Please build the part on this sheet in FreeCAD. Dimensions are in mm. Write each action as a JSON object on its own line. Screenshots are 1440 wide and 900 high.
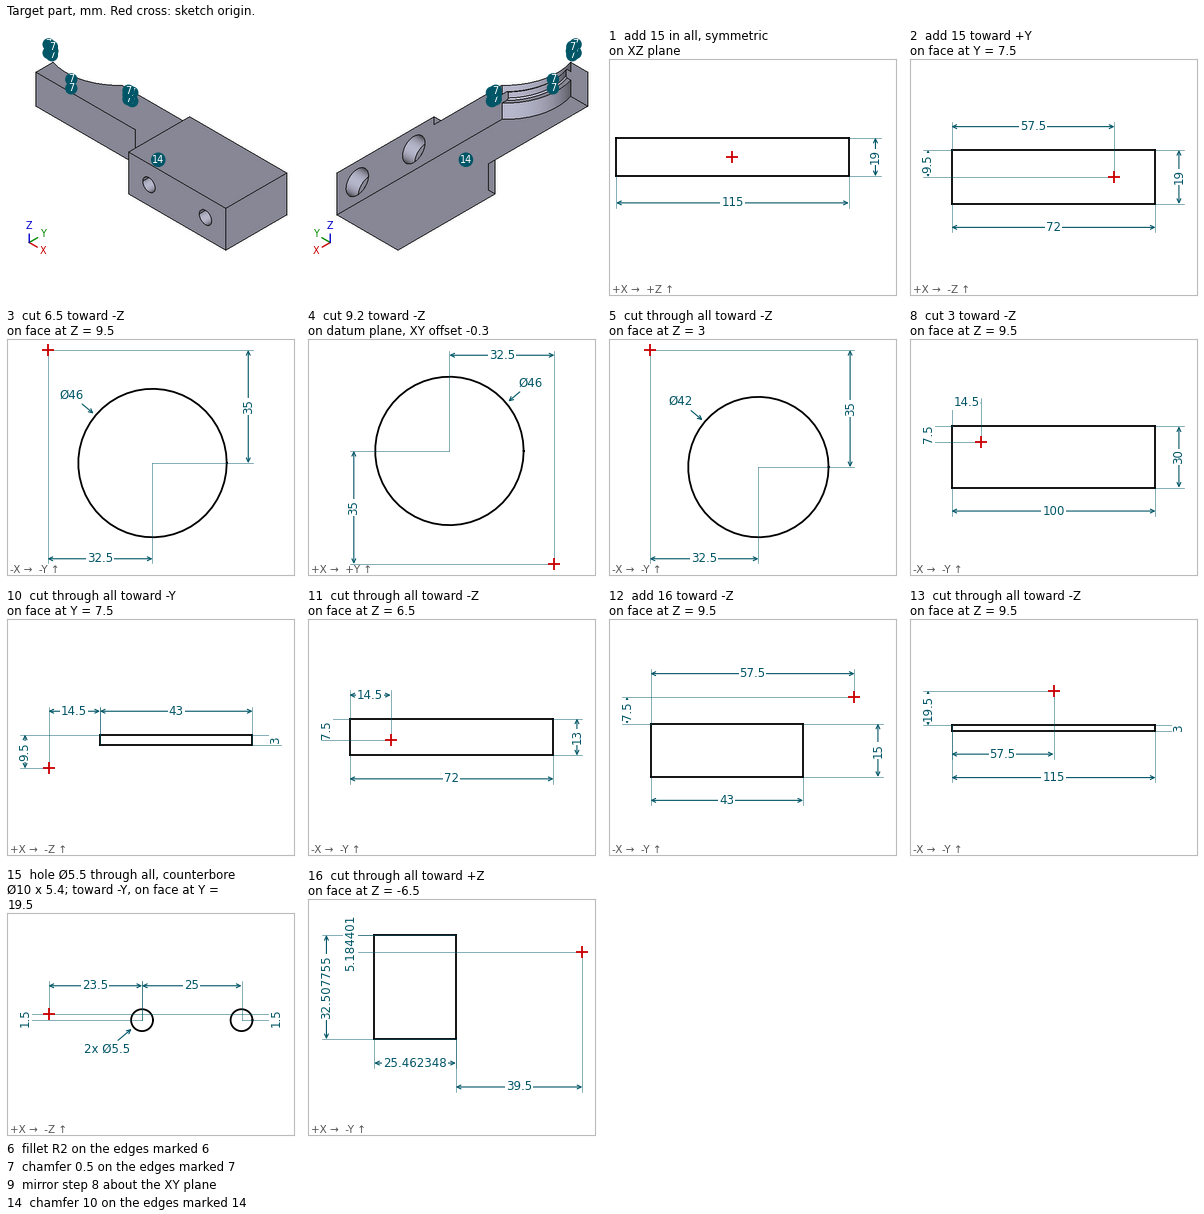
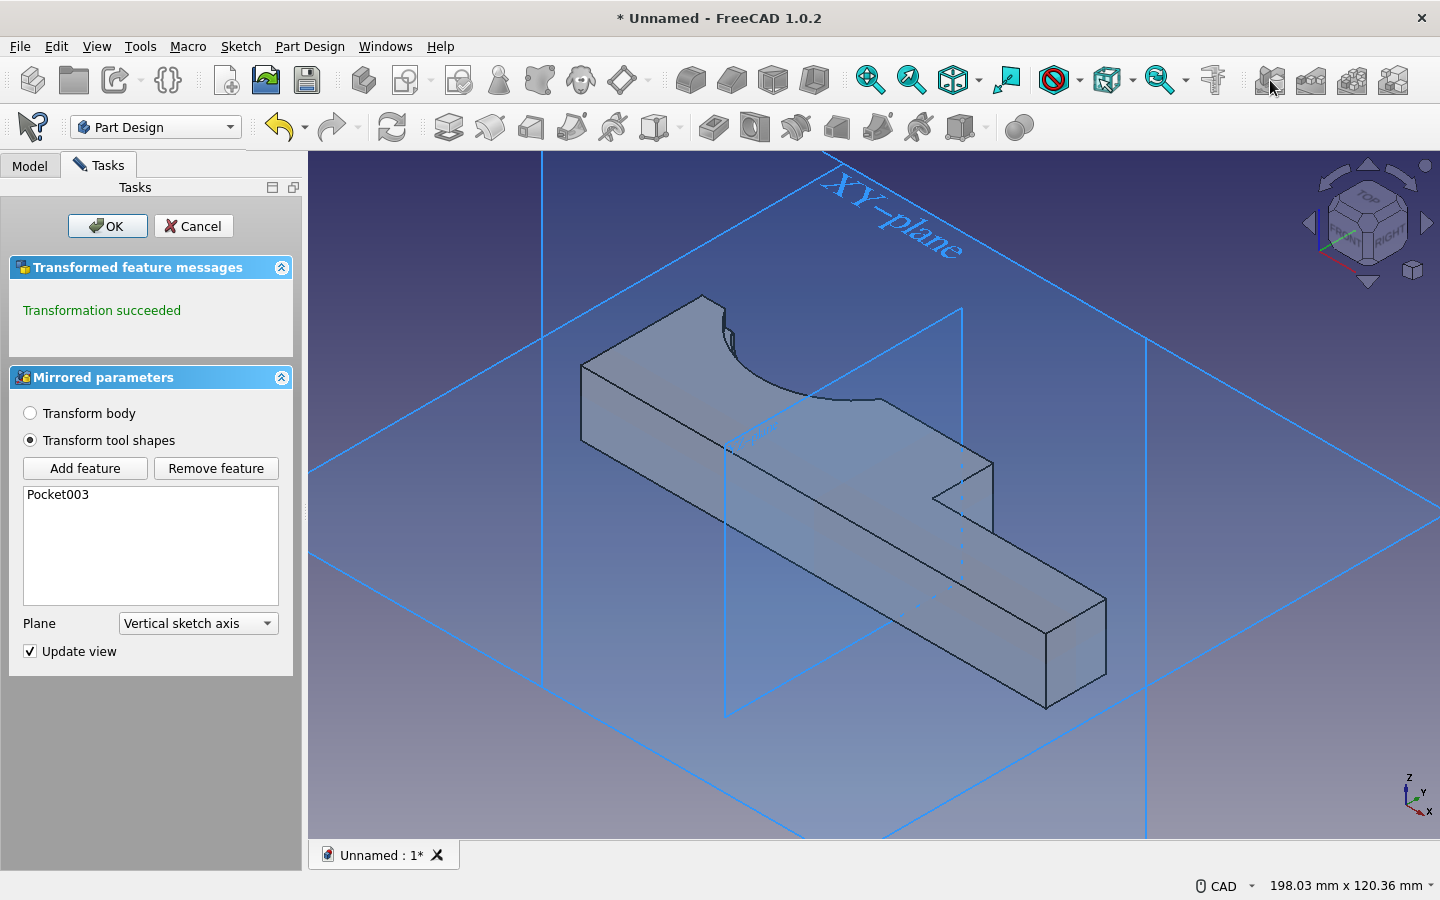
{"action": "left_click", "coordinate": [199, 624]}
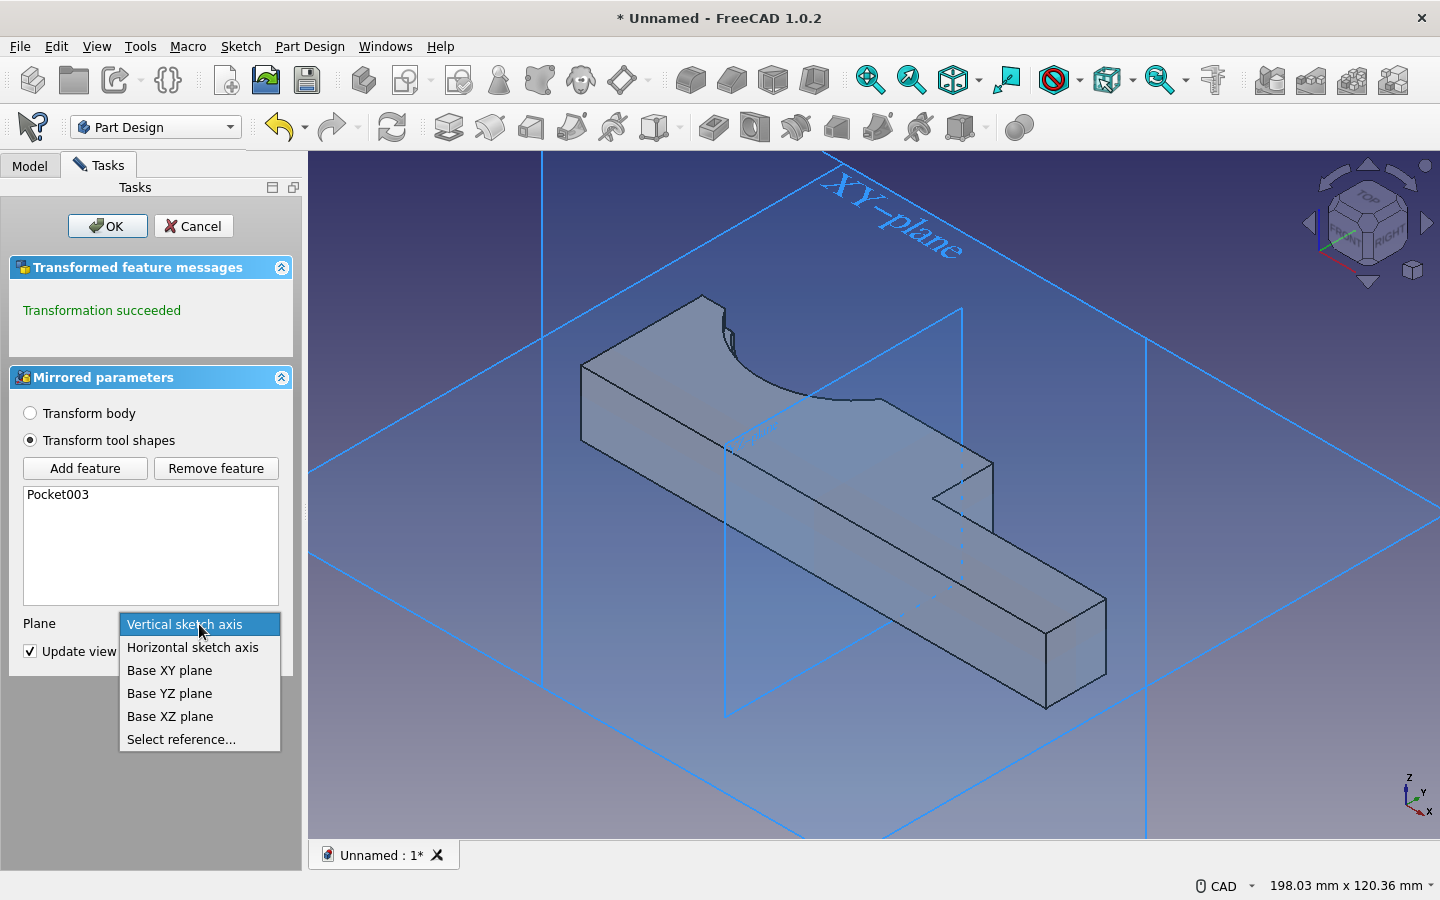
{"action": "left_click", "coordinate": [198, 670]}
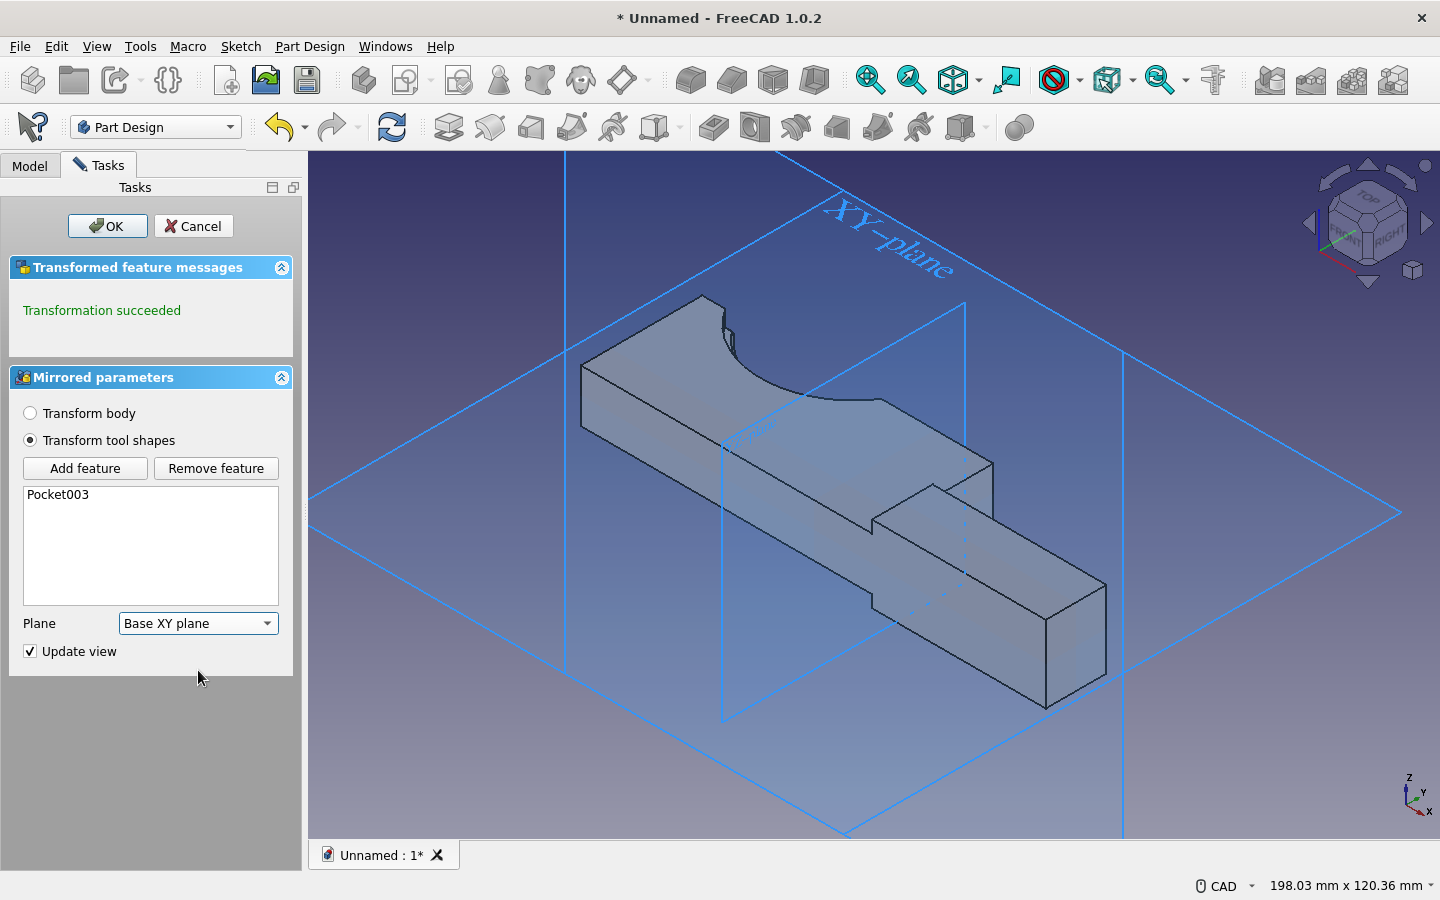
{"action": "left_click", "coordinate": [108, 226]}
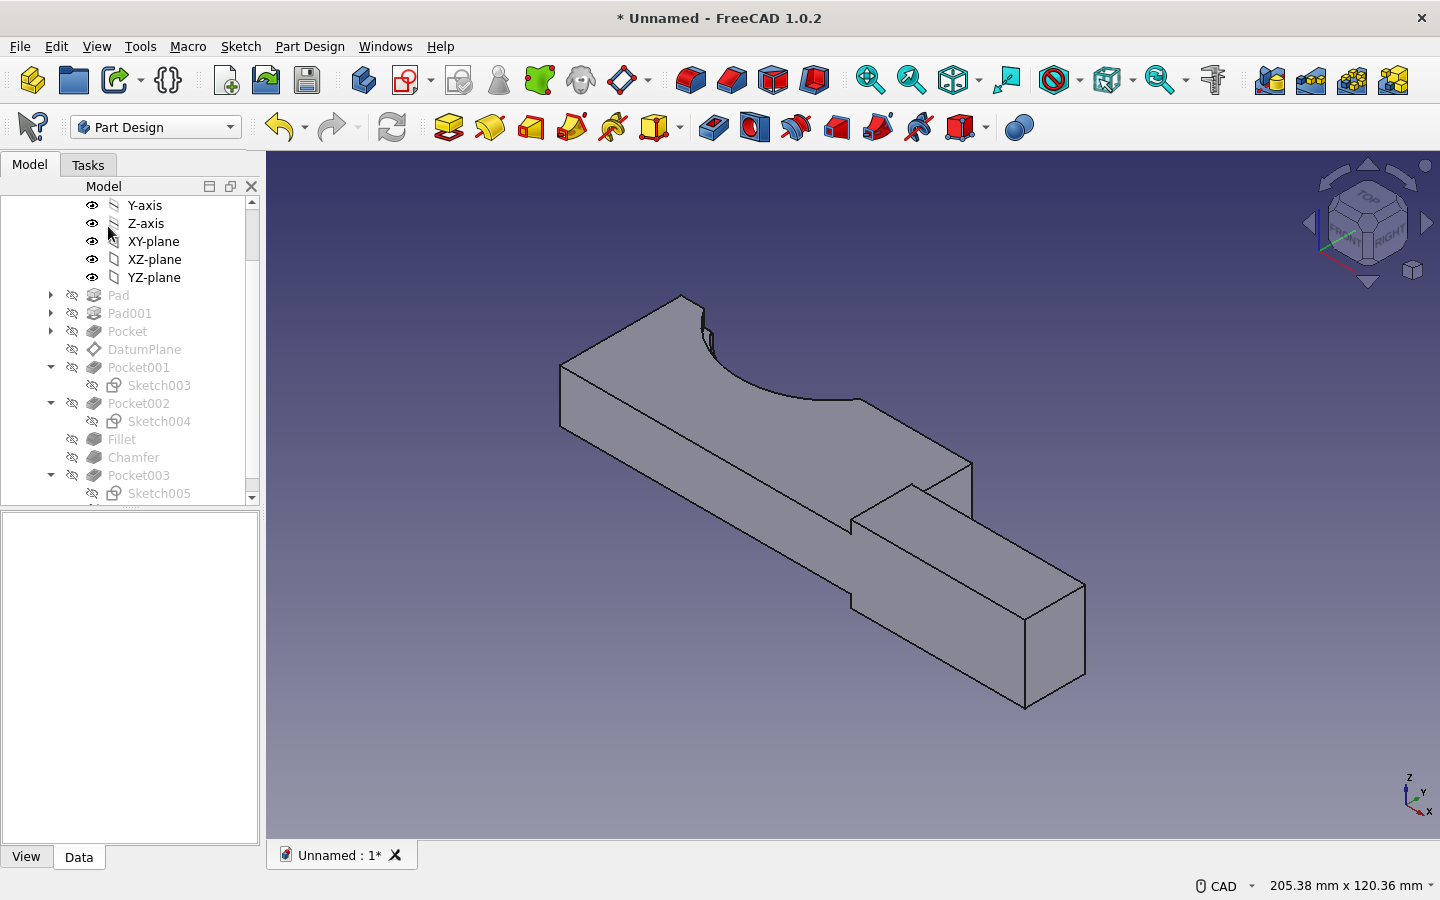
{"action": "key", "text": "4"}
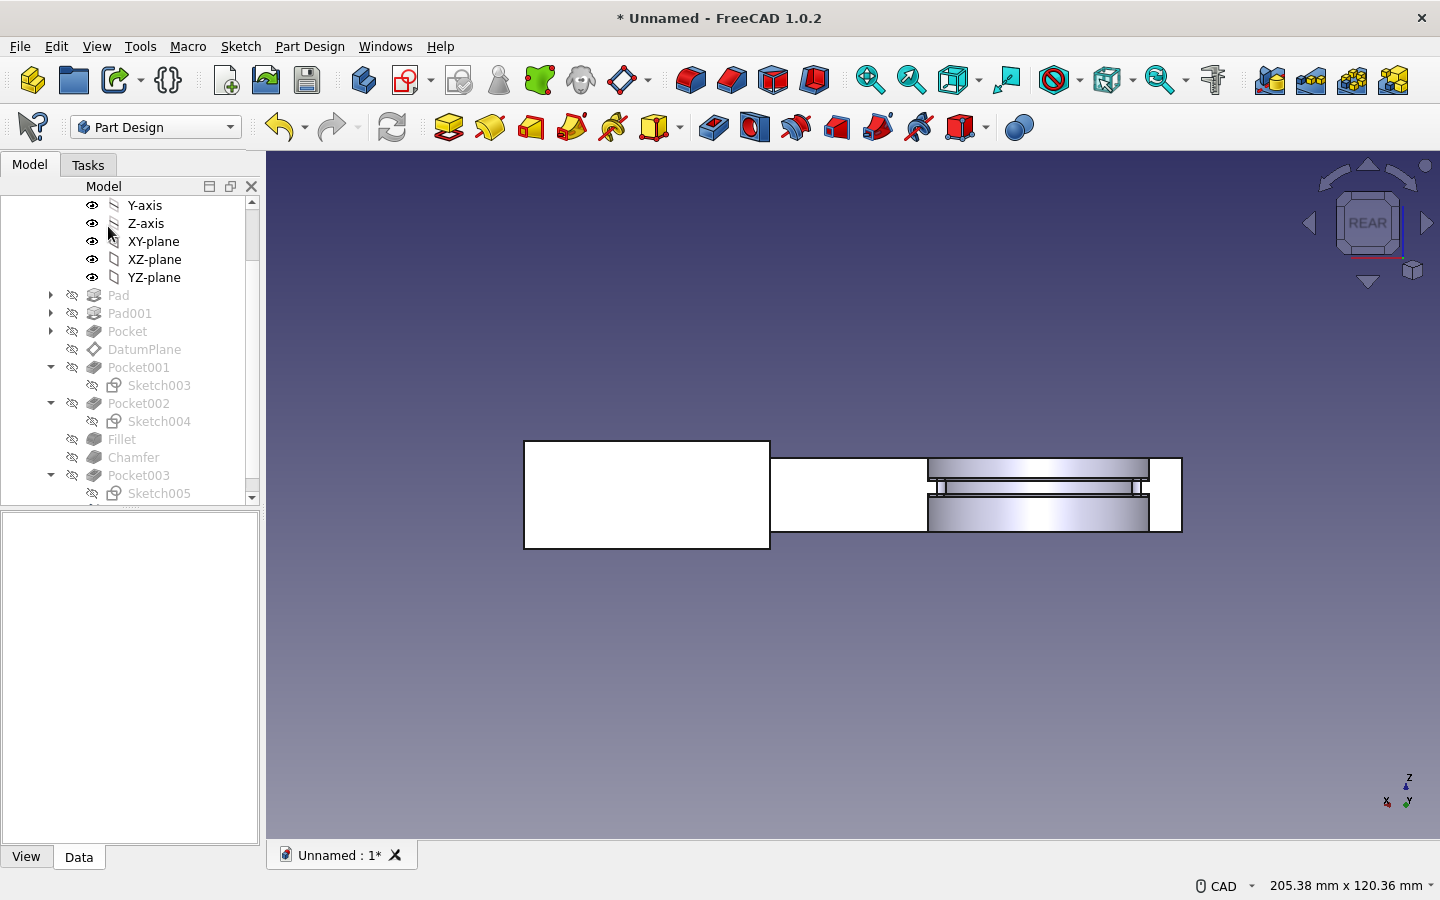
{"action": "left_click", "coordinate": [612, 494]}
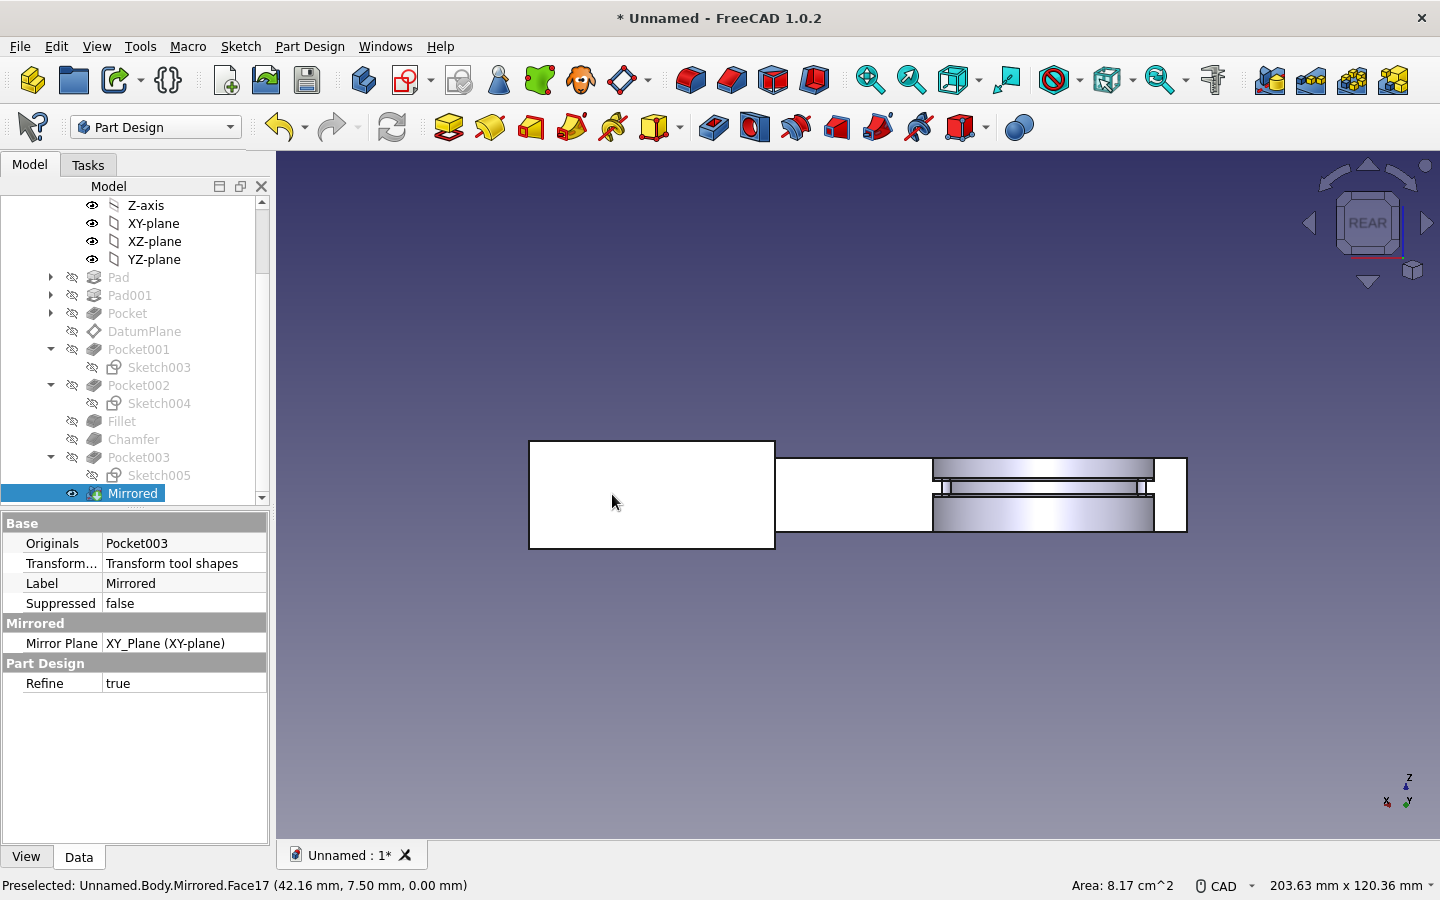
{"action": "left_click", "coordinate": [404, 80]}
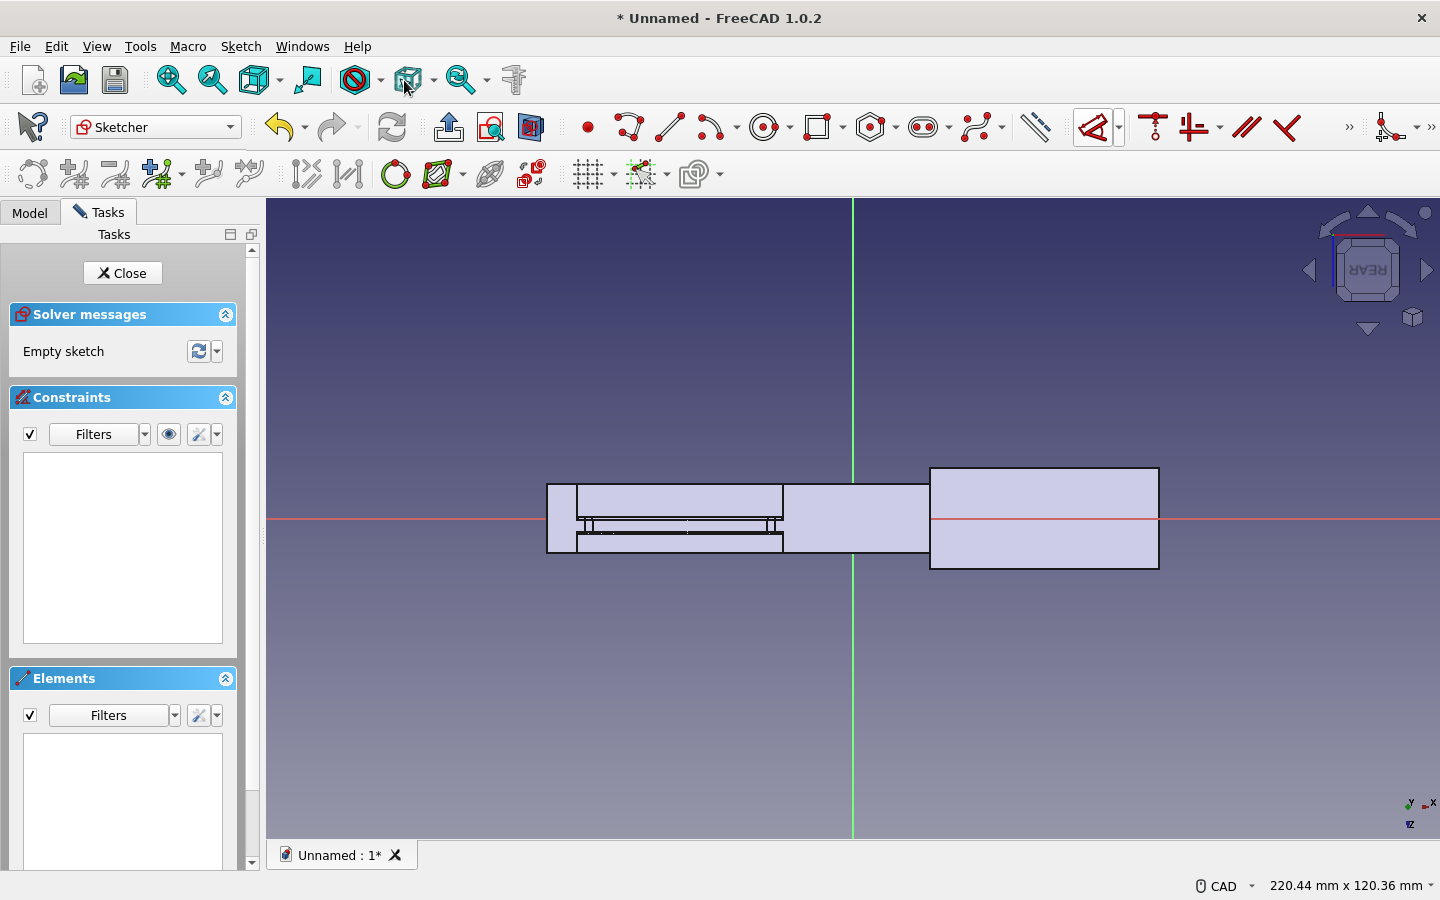
{"action": "scroll", "coordinate": [1187, 473], "scroll_direction": "up", "scroll_amount": 4}